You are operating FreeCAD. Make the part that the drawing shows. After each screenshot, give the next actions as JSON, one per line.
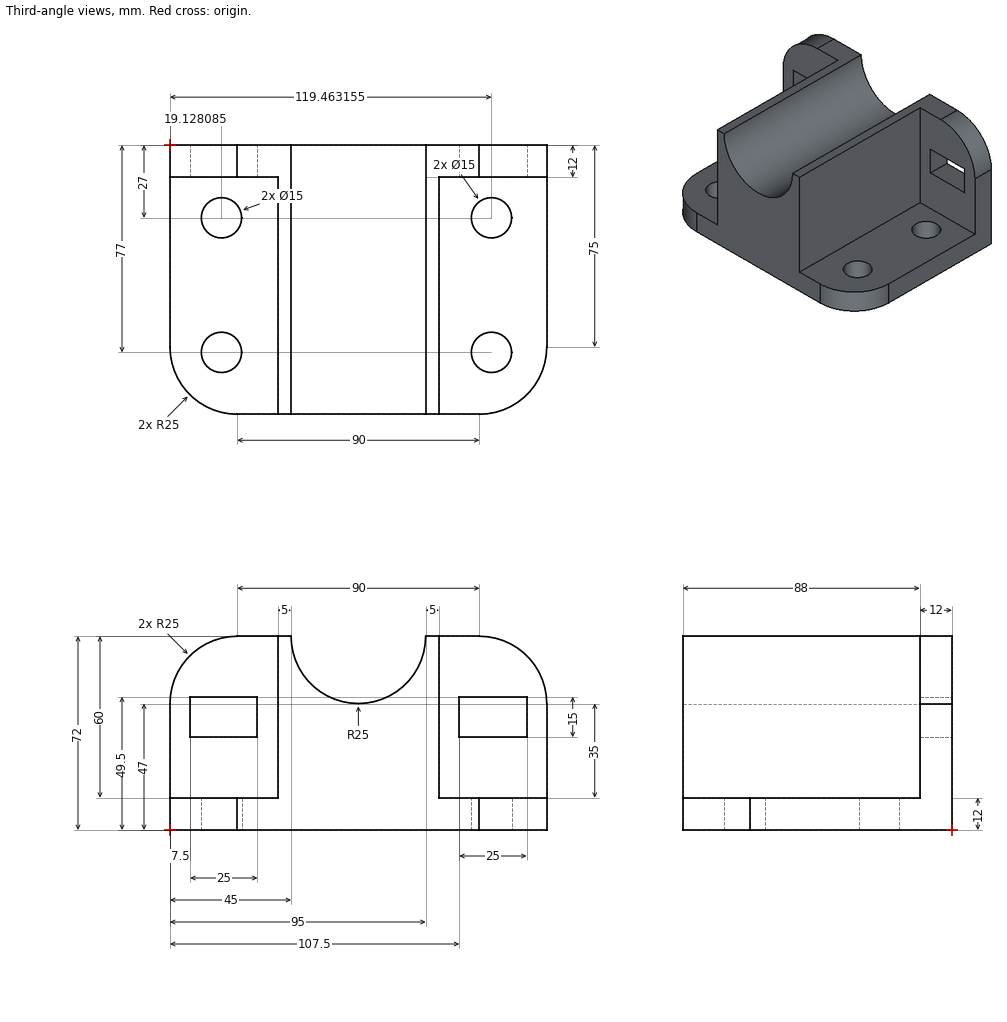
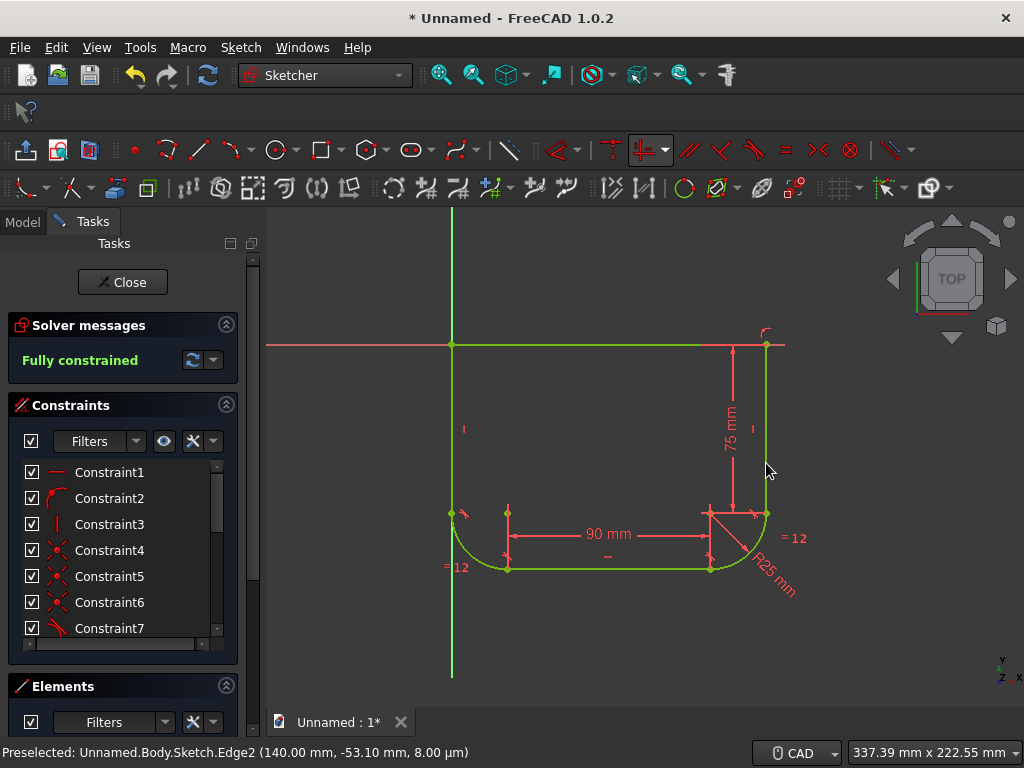
{"action": "left_click", "coordinate": [123, 282]}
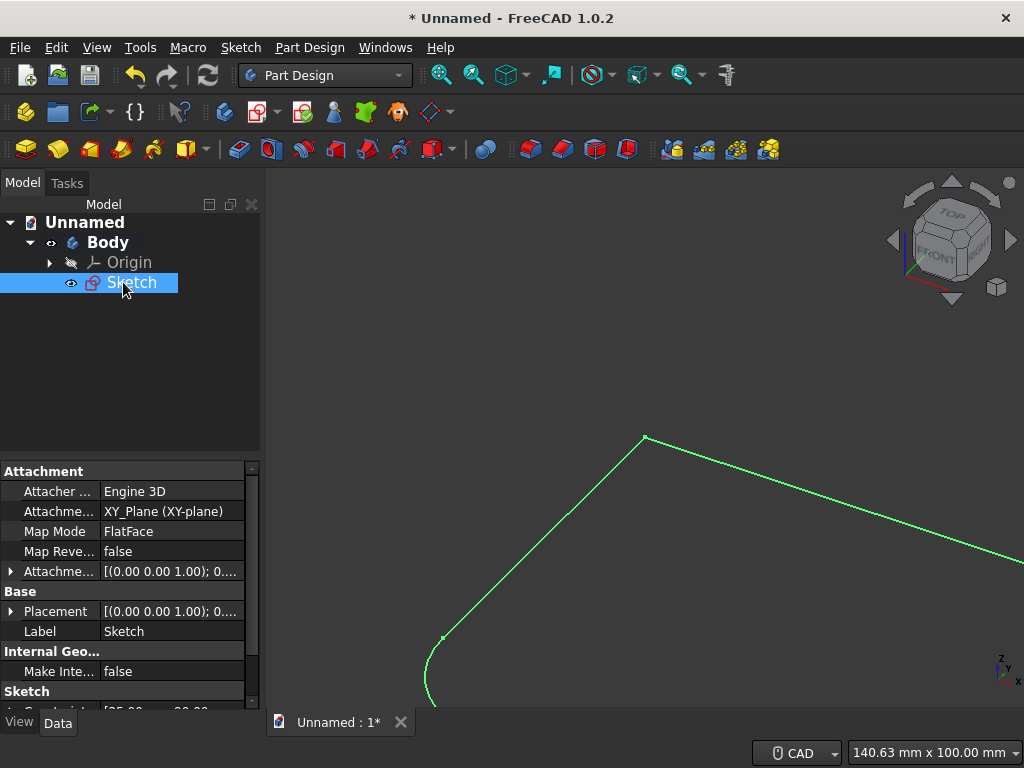
{"action": "left_click", "coordinate": [26, 150]}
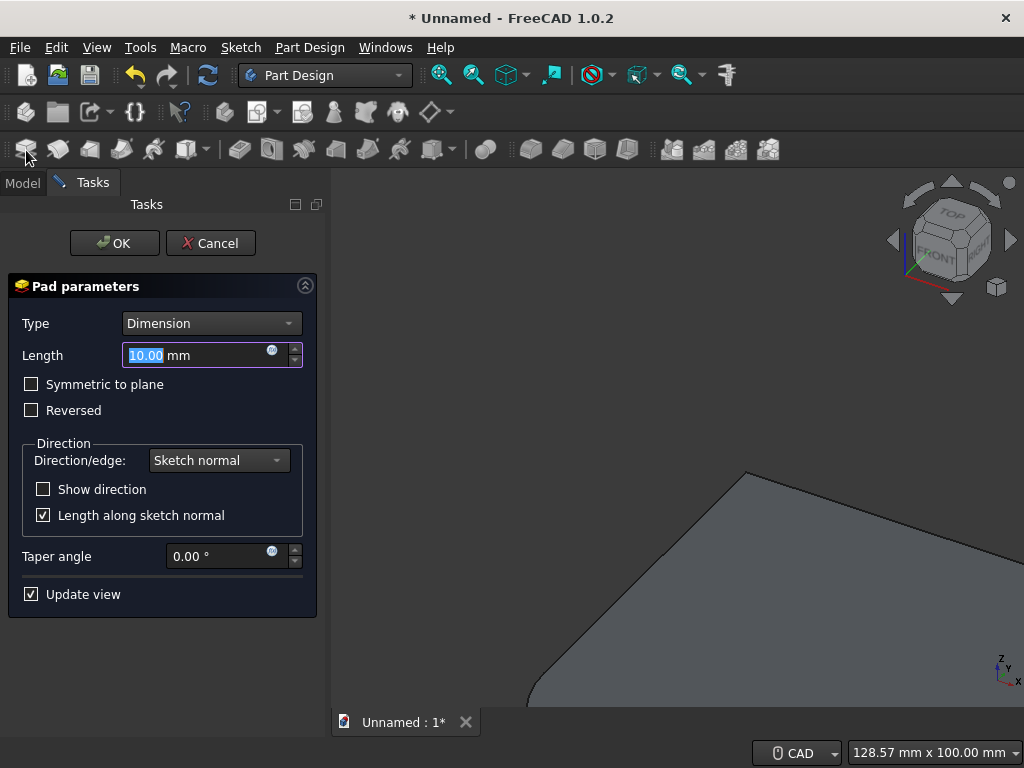
{"action": "type", "text": "12"}
{"action": "key", "text": "Tab"}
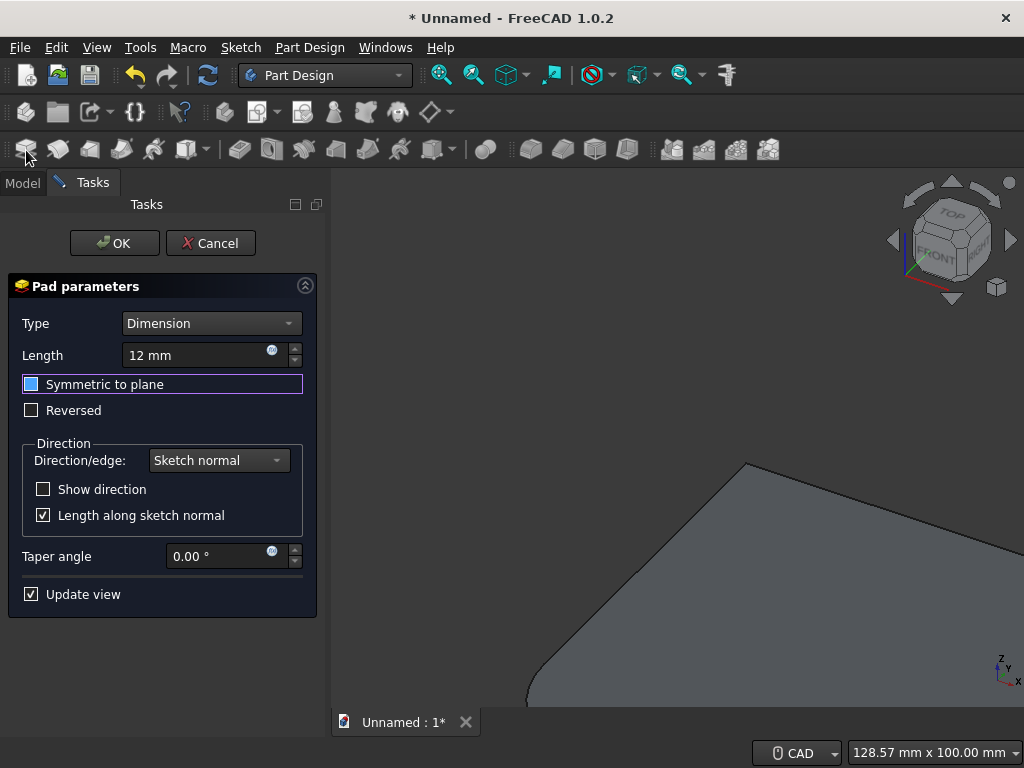
{"action": "left_click", "coordinate": [115, 243]}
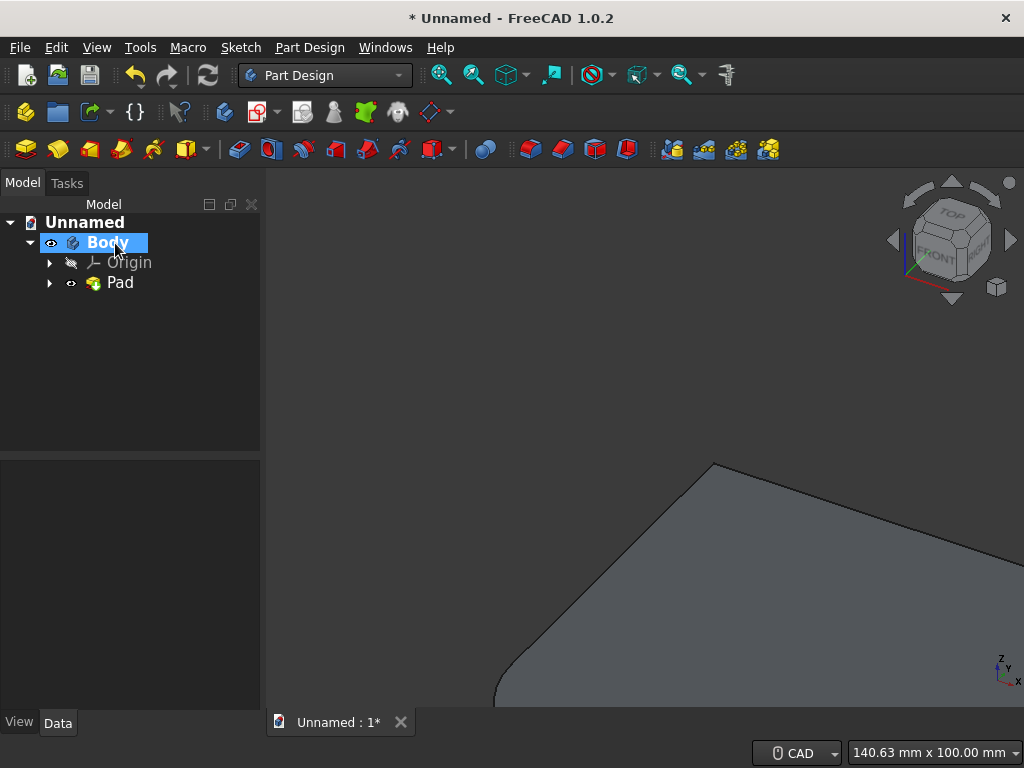
{"action": "key", "text": "v f"}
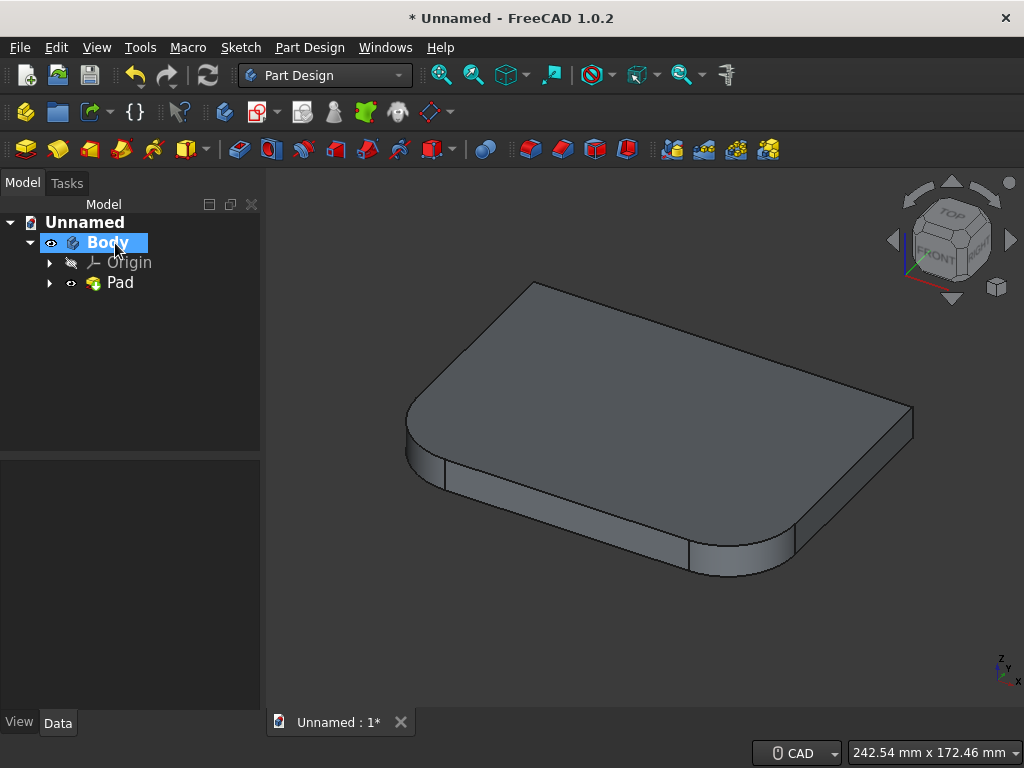
{"action": "key", "text": "4"}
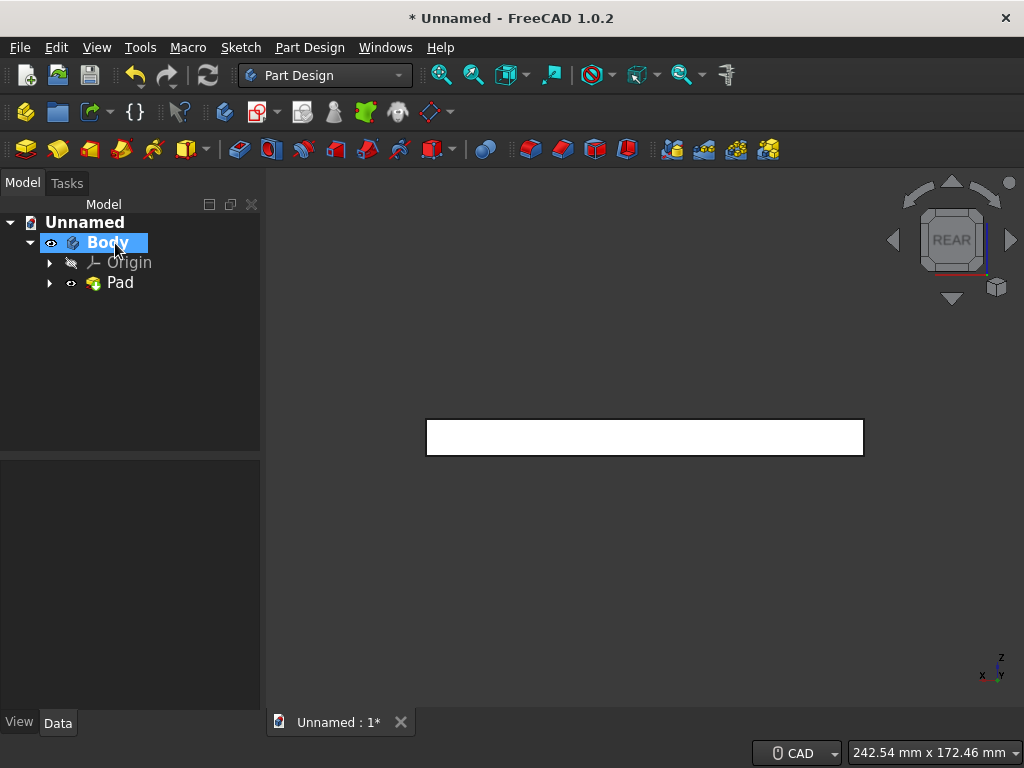
{"action": "left_click", "coordinate": [457, 436]}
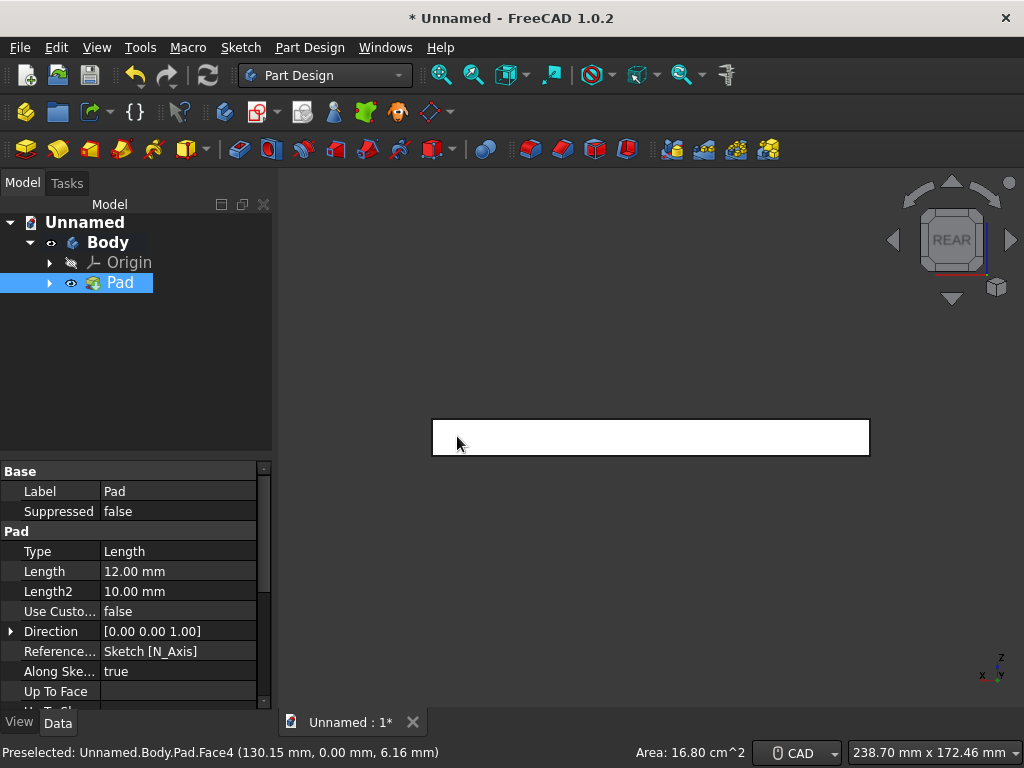
{"action": "left_click", "coordinate": [258, 112]}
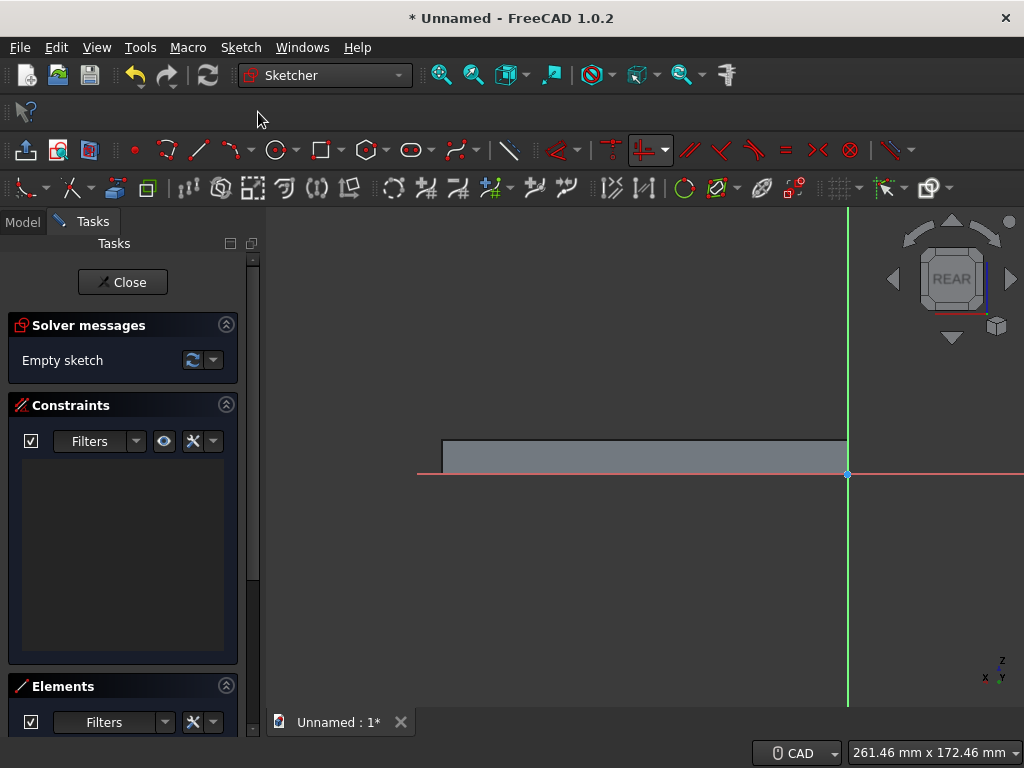
{"action": "scroll", "coordinate": [294, 679], "scroll_direction": "down", "scroll_amount": 1}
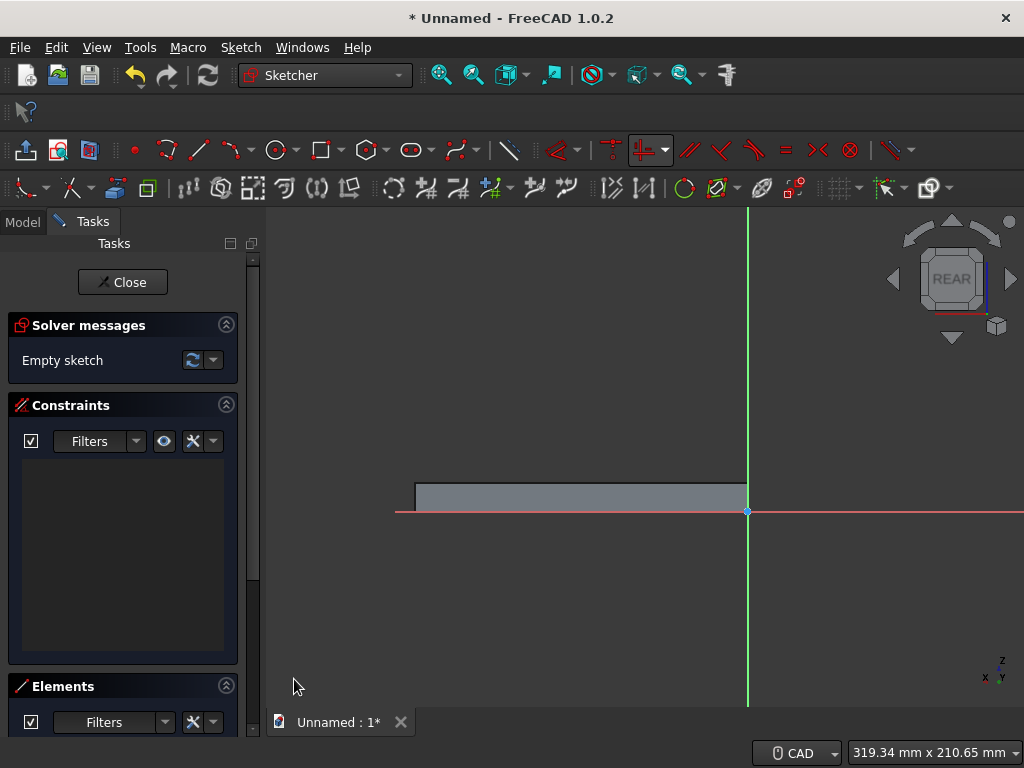
{"action": "key", "text": "g m"}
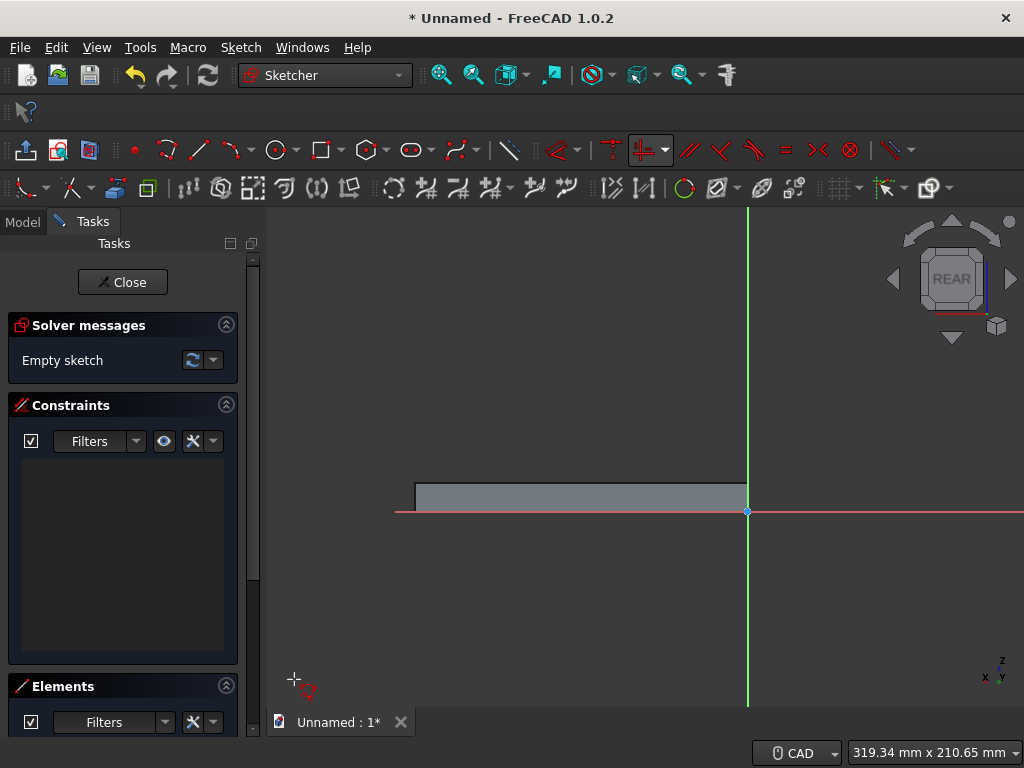
{"action": "left_click", "coordinate": [415, 400]}
{"action": "left_click", "coordinate": [415, 483]}
{"action": "left_click", "coordinate": [748, 483]}
{"action": "left_click", "coordinate": [739, 400]}
{"action": "right_click", "coordinate": [739, 400]}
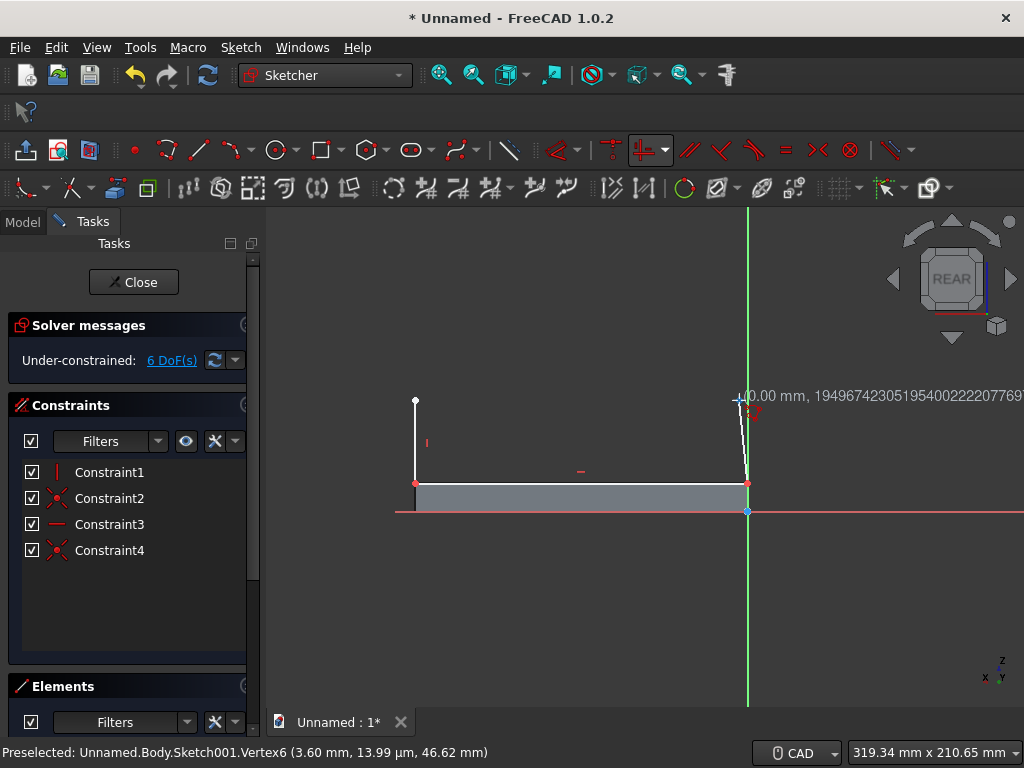
{"action": "key", "text": "g l"}